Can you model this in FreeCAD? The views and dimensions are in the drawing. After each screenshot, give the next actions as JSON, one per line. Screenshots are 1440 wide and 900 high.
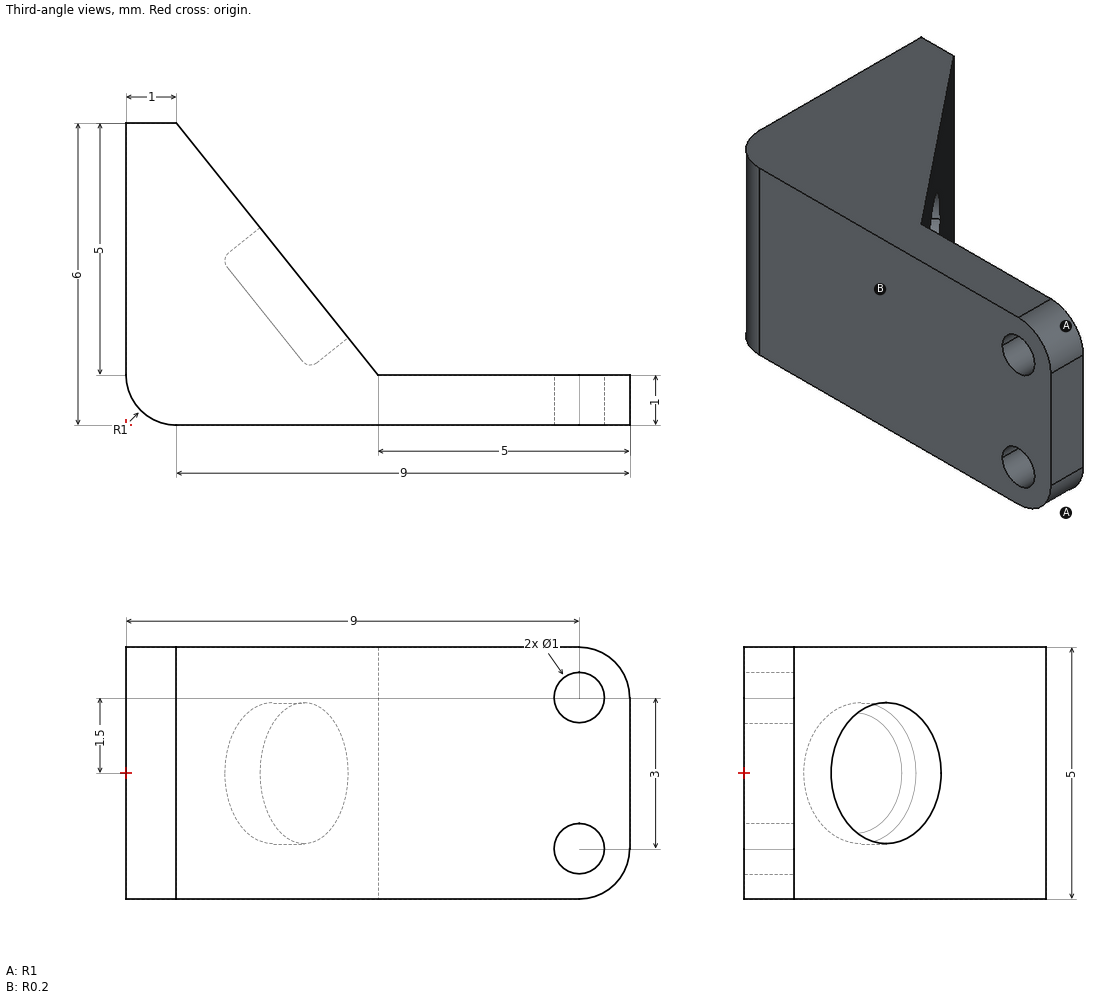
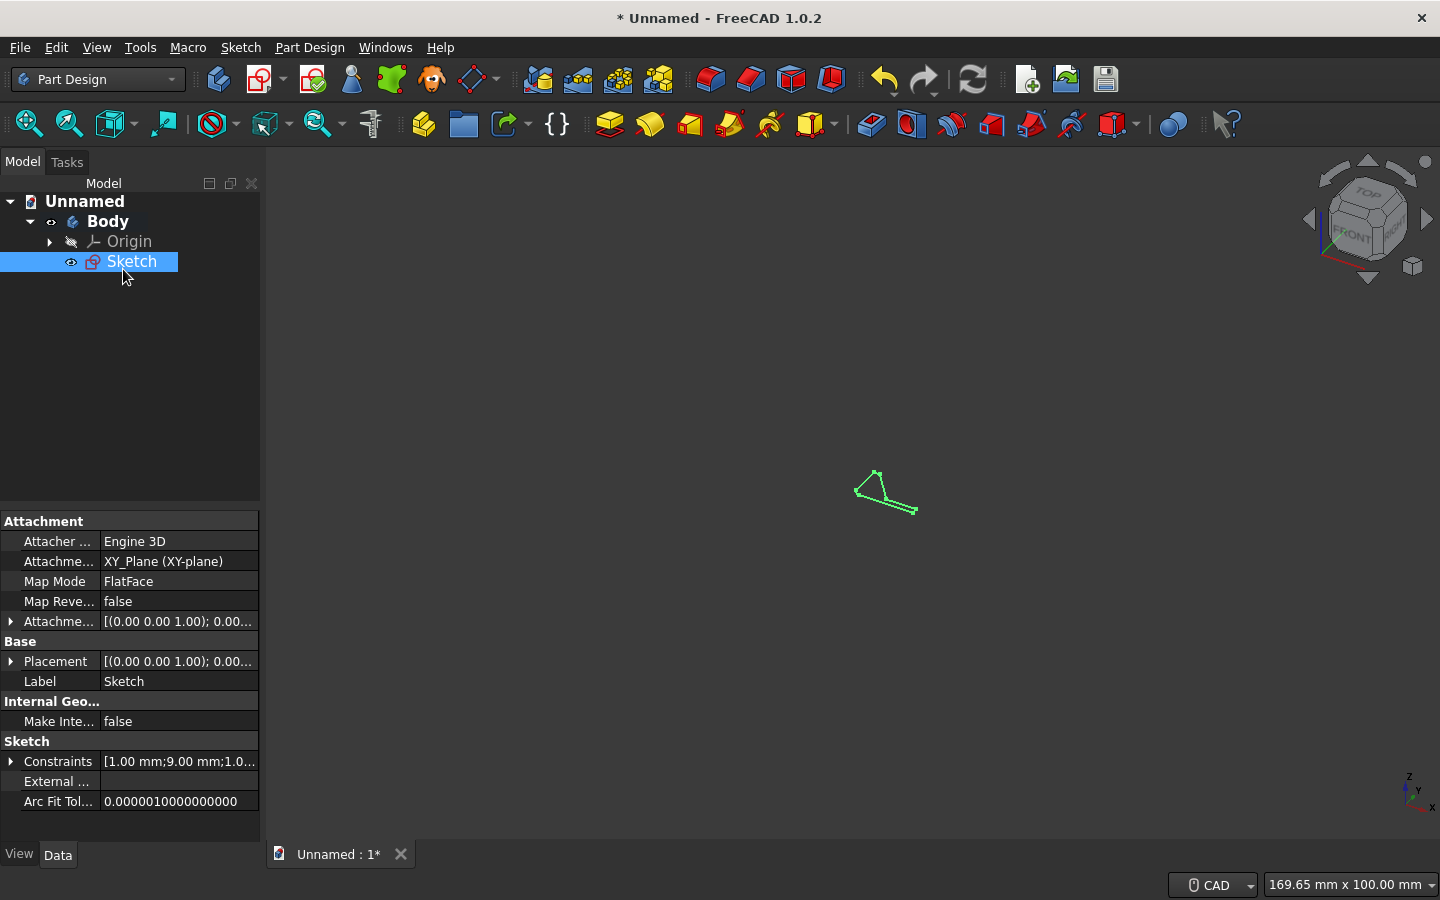
{"action": "left_click", "coordinate": [610, 124]}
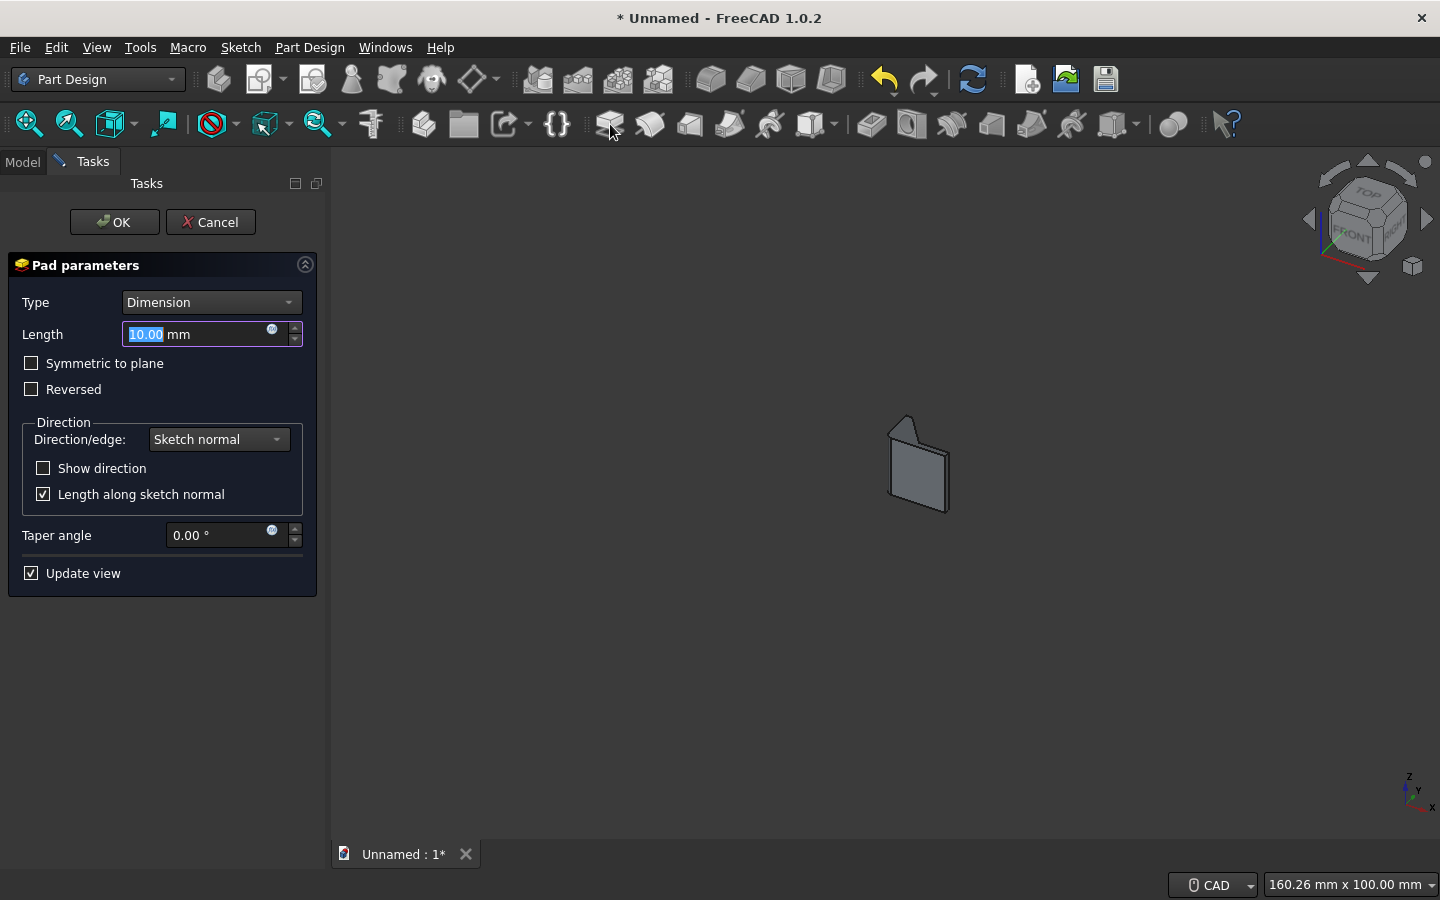
{"action": "type", "text": "5"}
{"action": "key", "text": "Tab"}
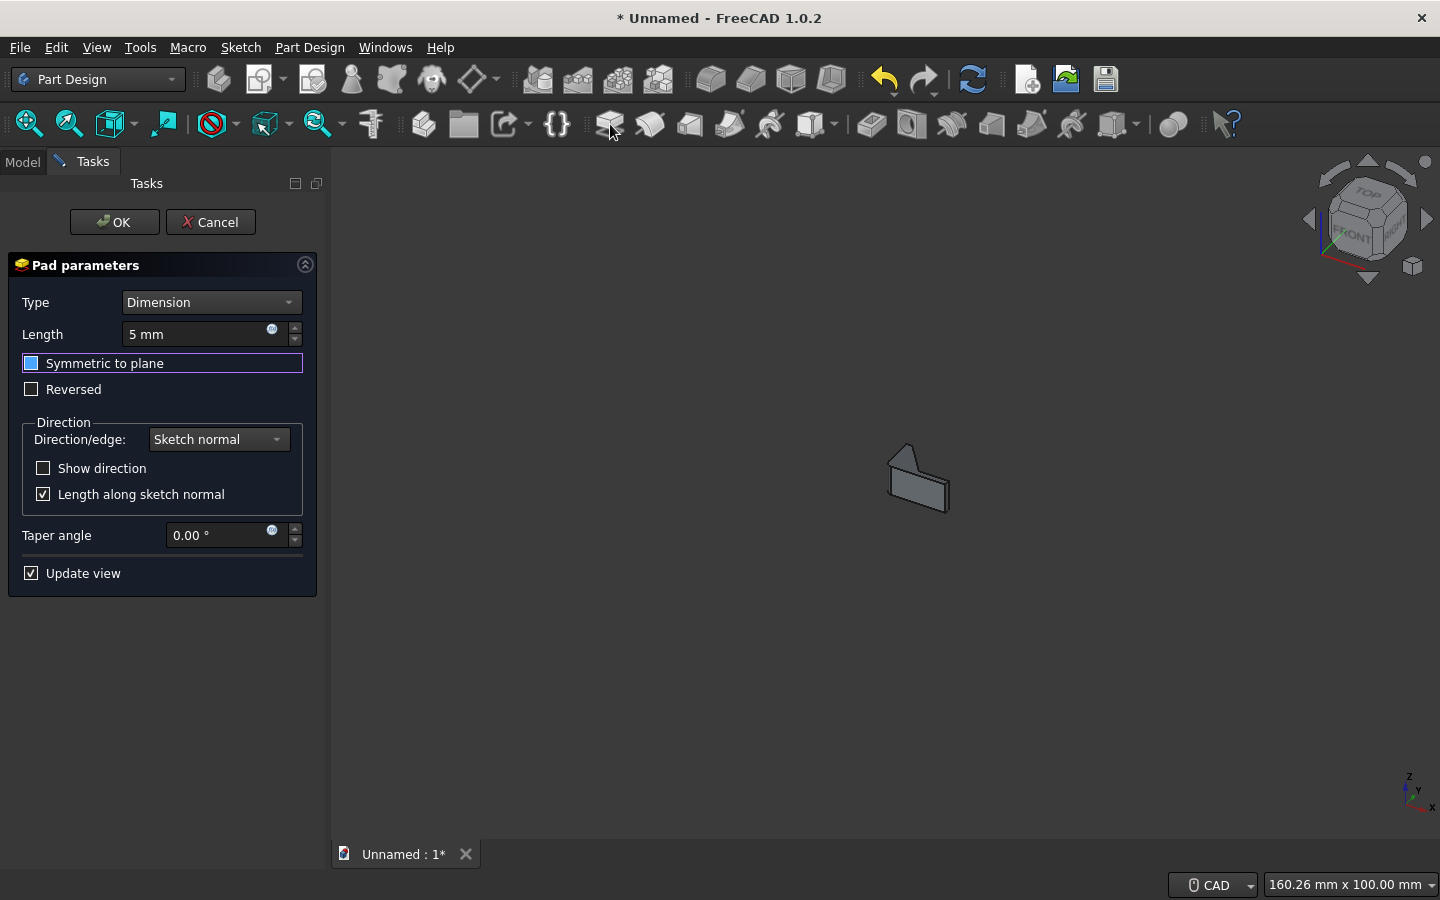
{"action": "left_click", "coordinate": [30, 363]}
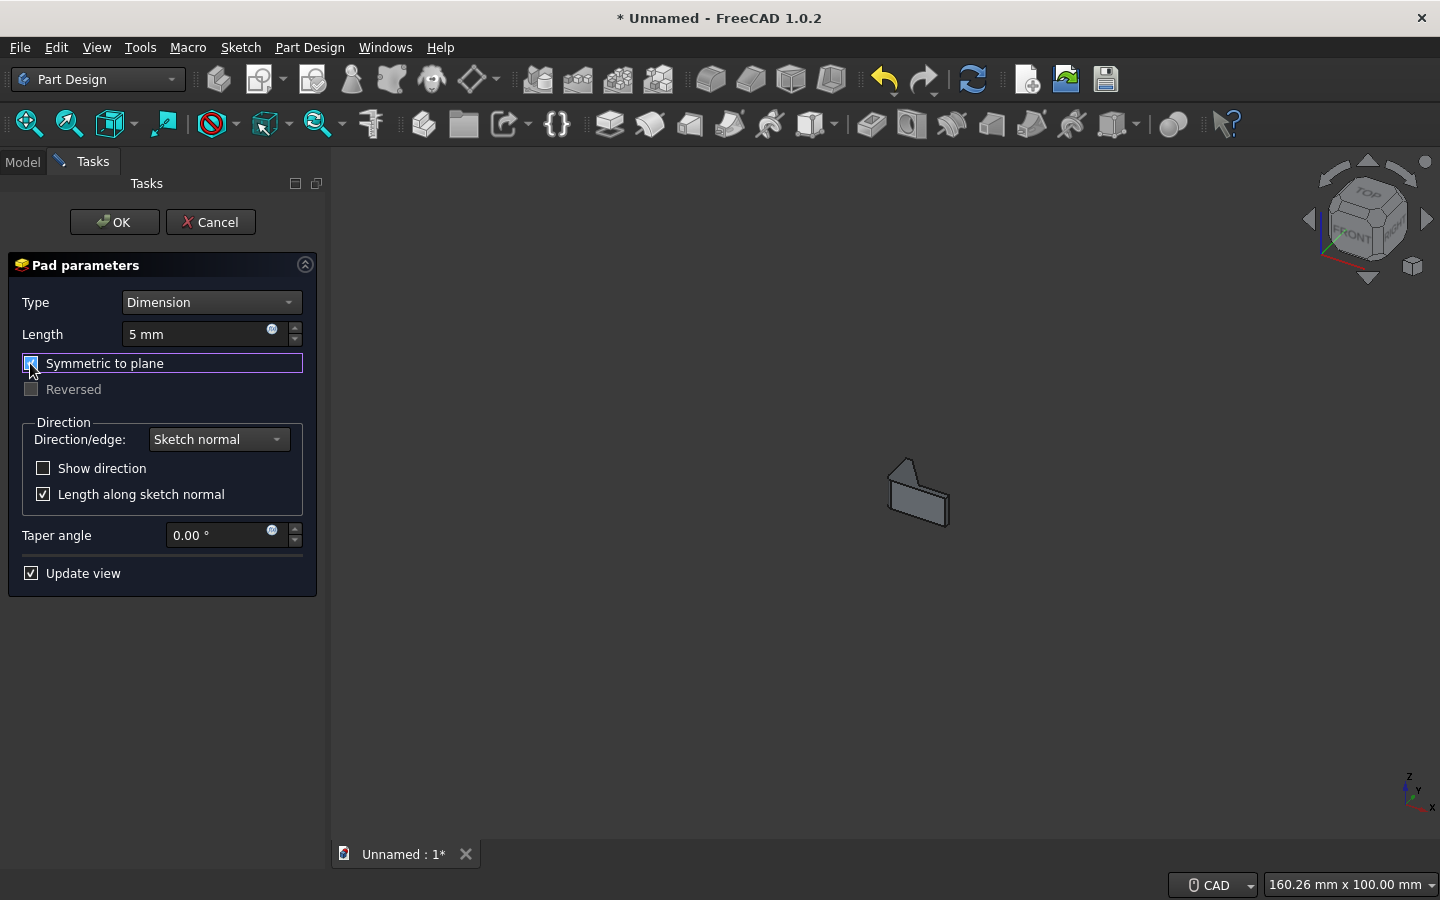
{"action": "left_click", "coordinate": [115, 222]}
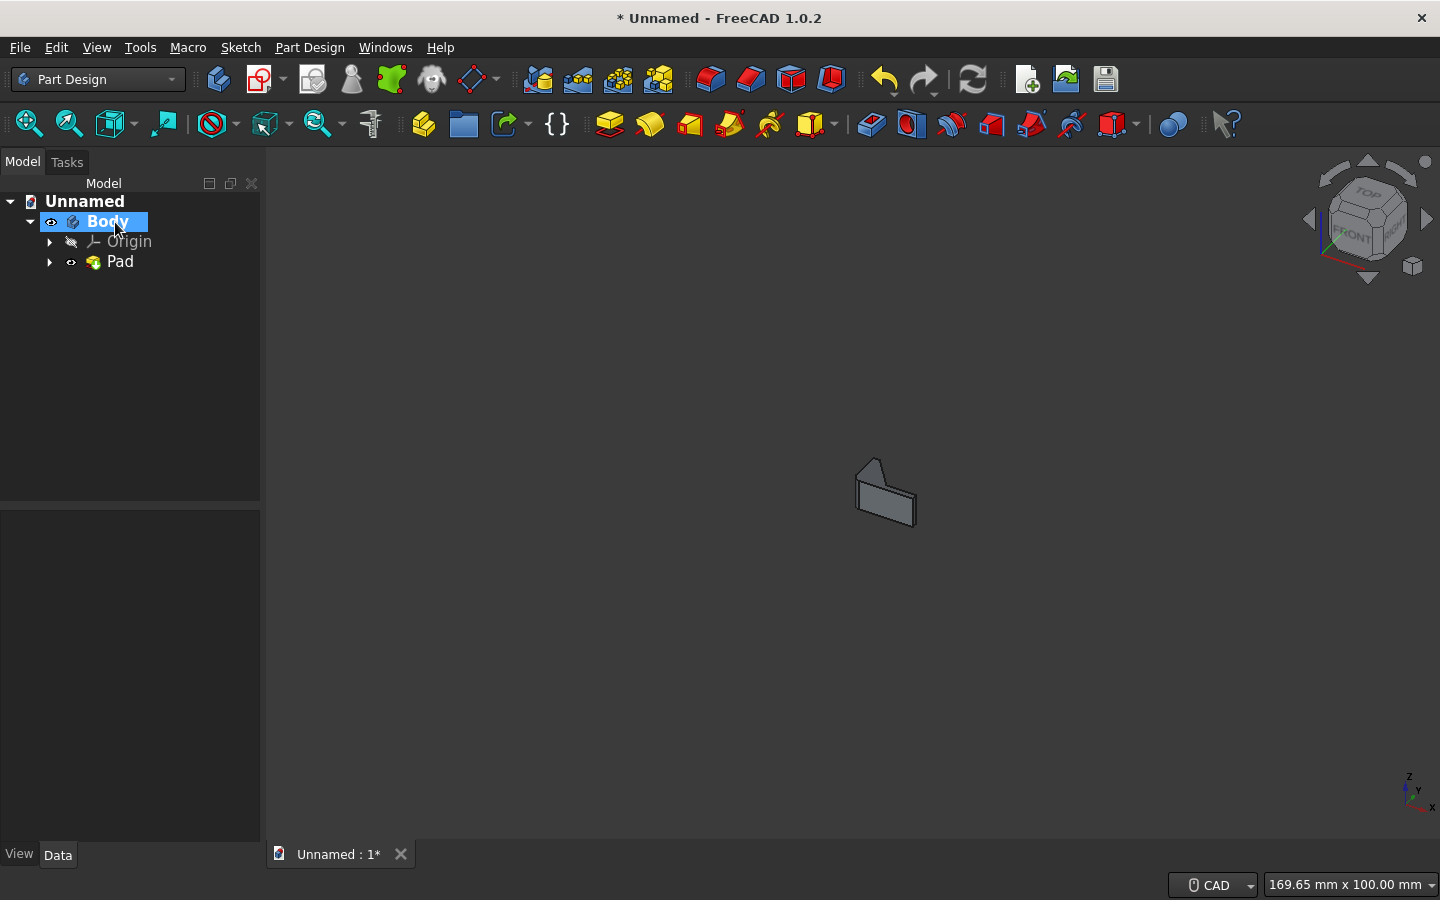
{"action": "left_click", "coordinate": [30, 124]}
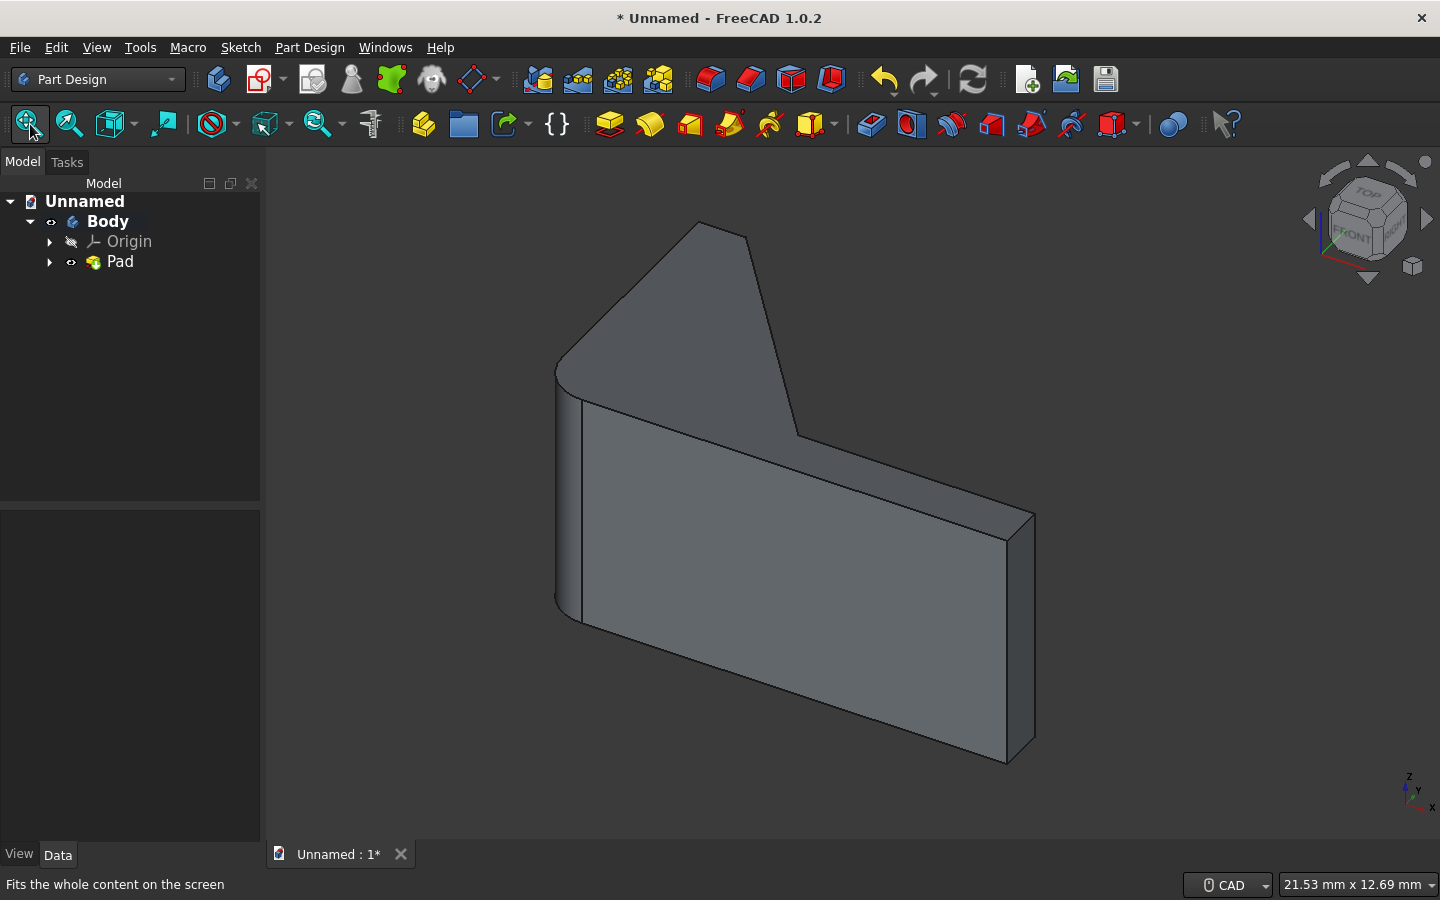
{"action": "key", "text": "3"}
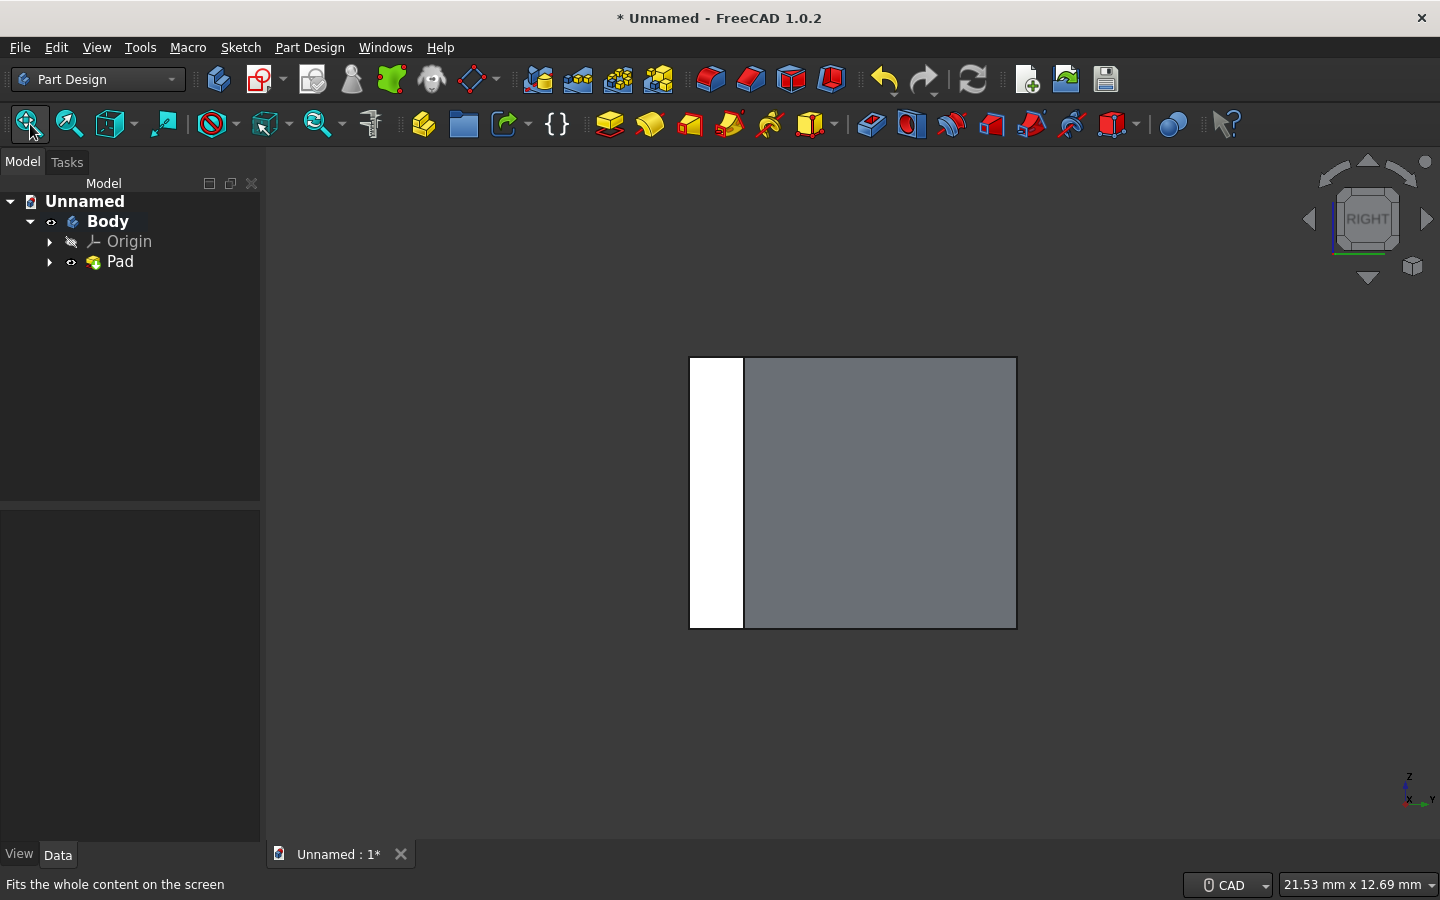
{"action": "left_click", "coordinate": [30, 124]}